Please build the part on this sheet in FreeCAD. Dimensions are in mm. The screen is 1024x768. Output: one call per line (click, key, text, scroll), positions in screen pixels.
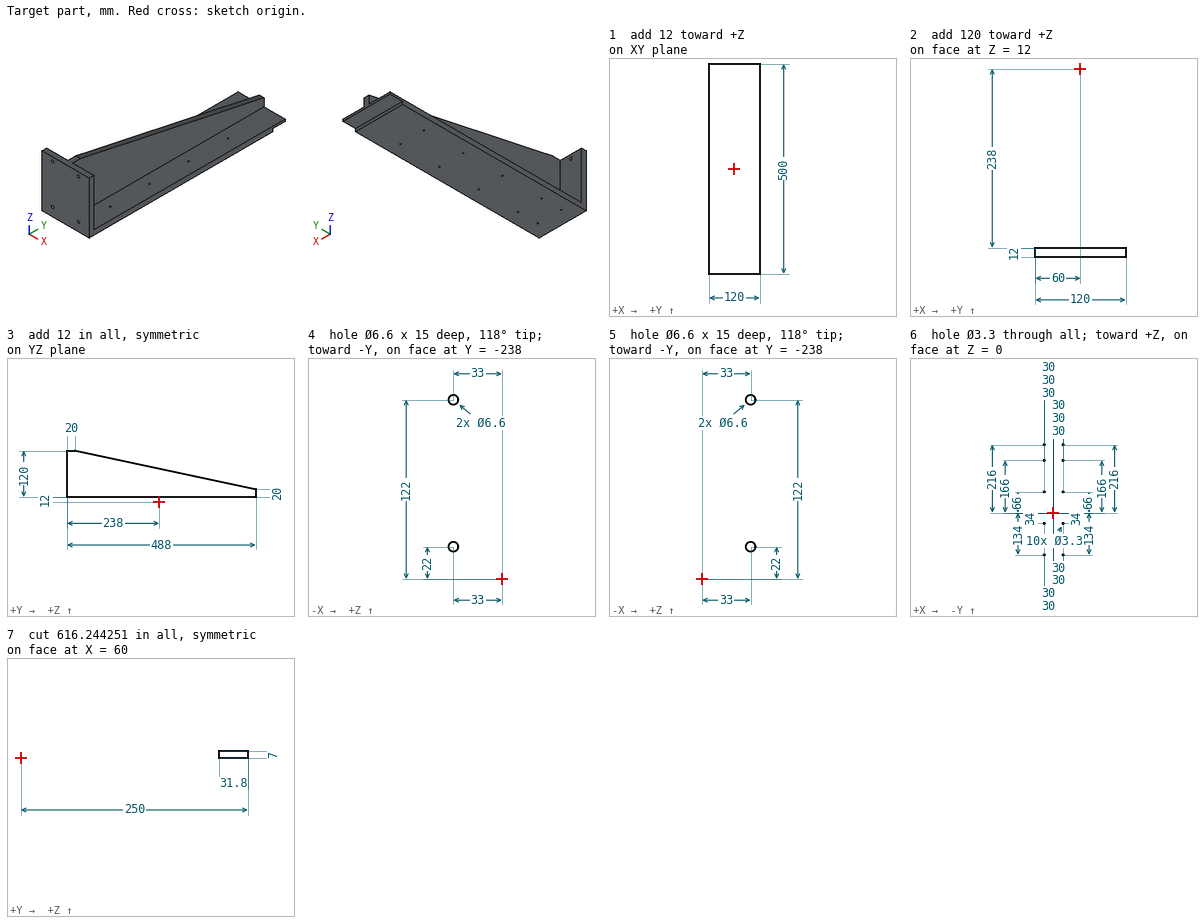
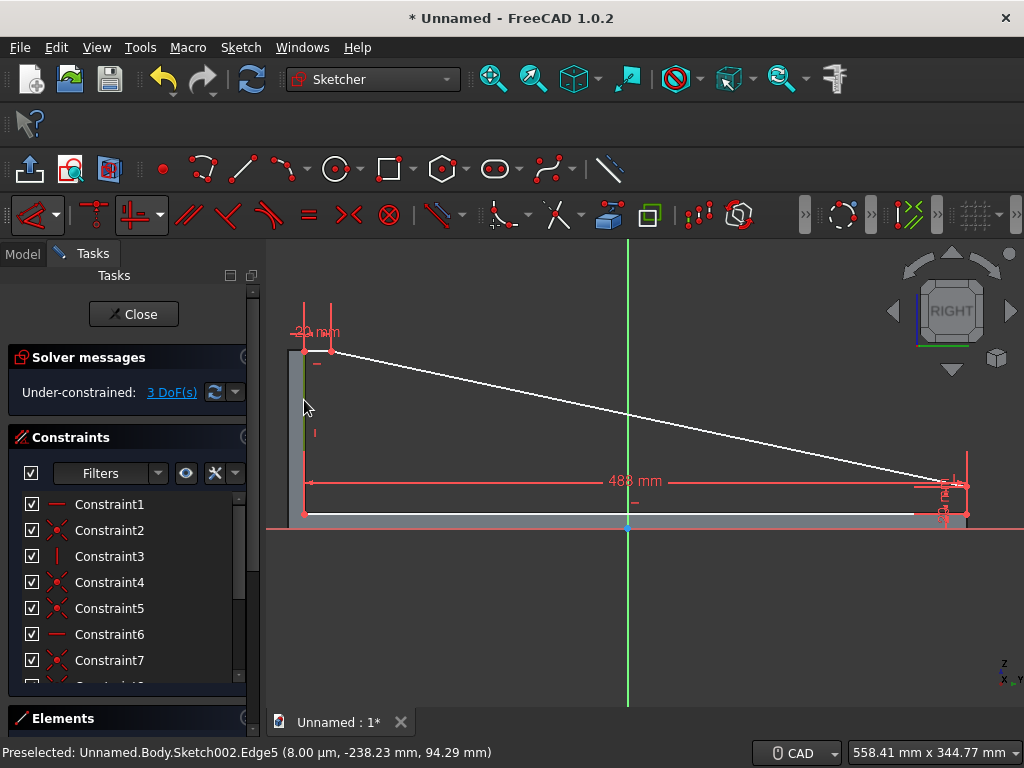
click(58, 216)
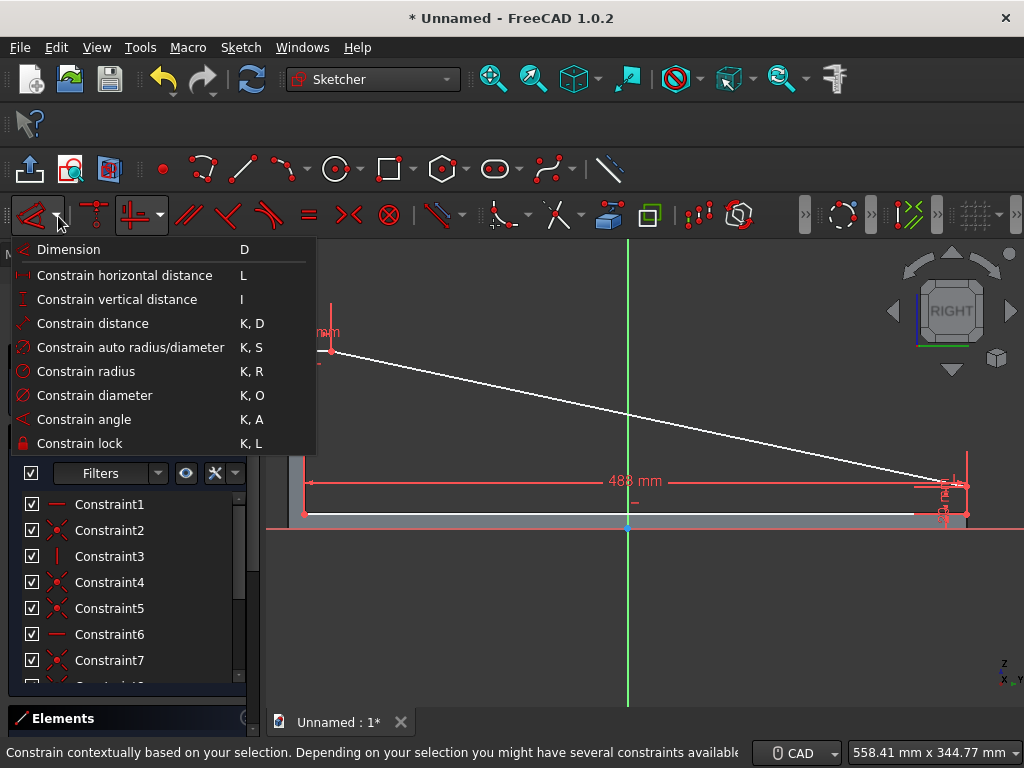
click(164, 299)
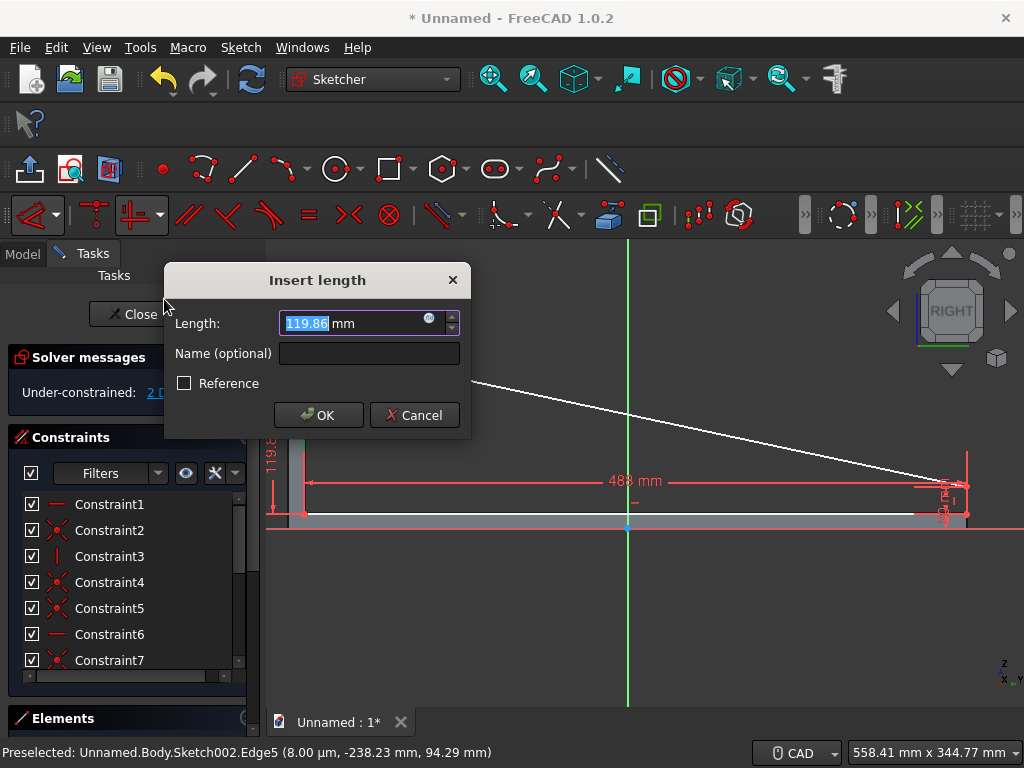
text(120)
key(Return)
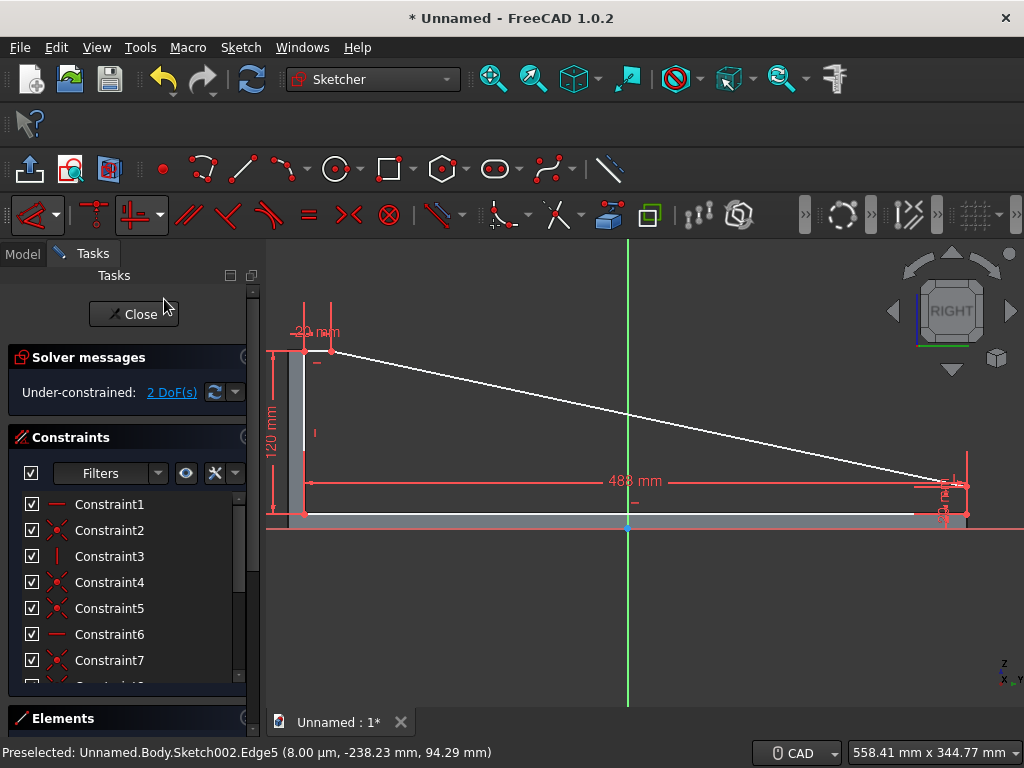
scroll(304, 514, up, 5)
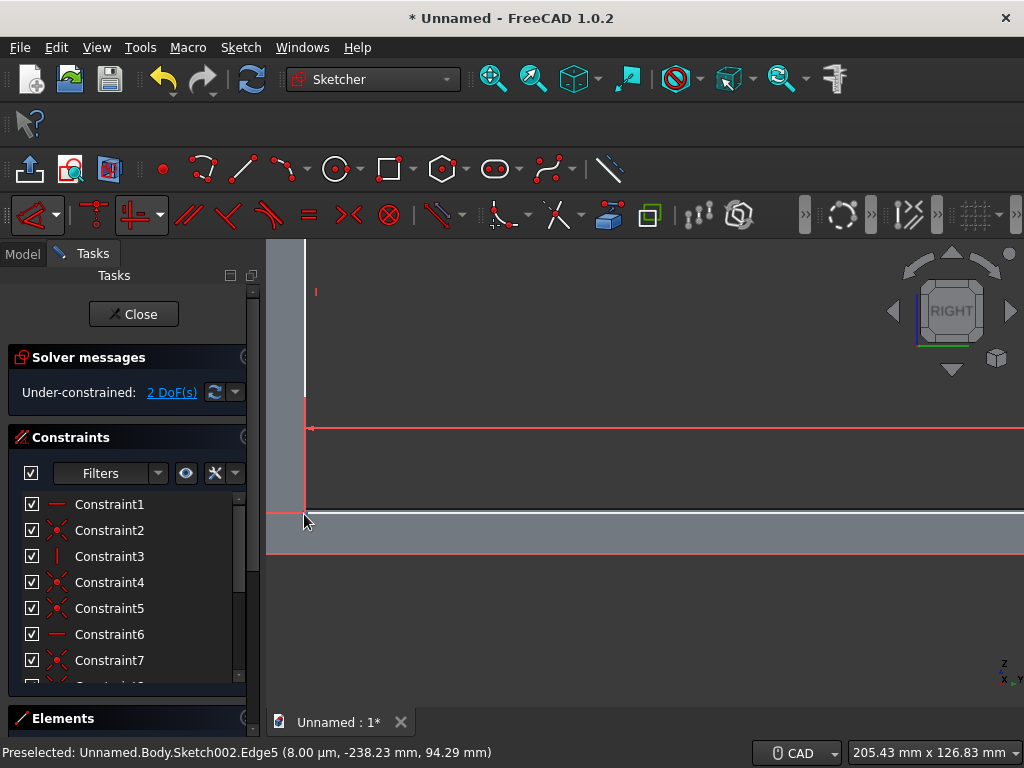
click(305, 513)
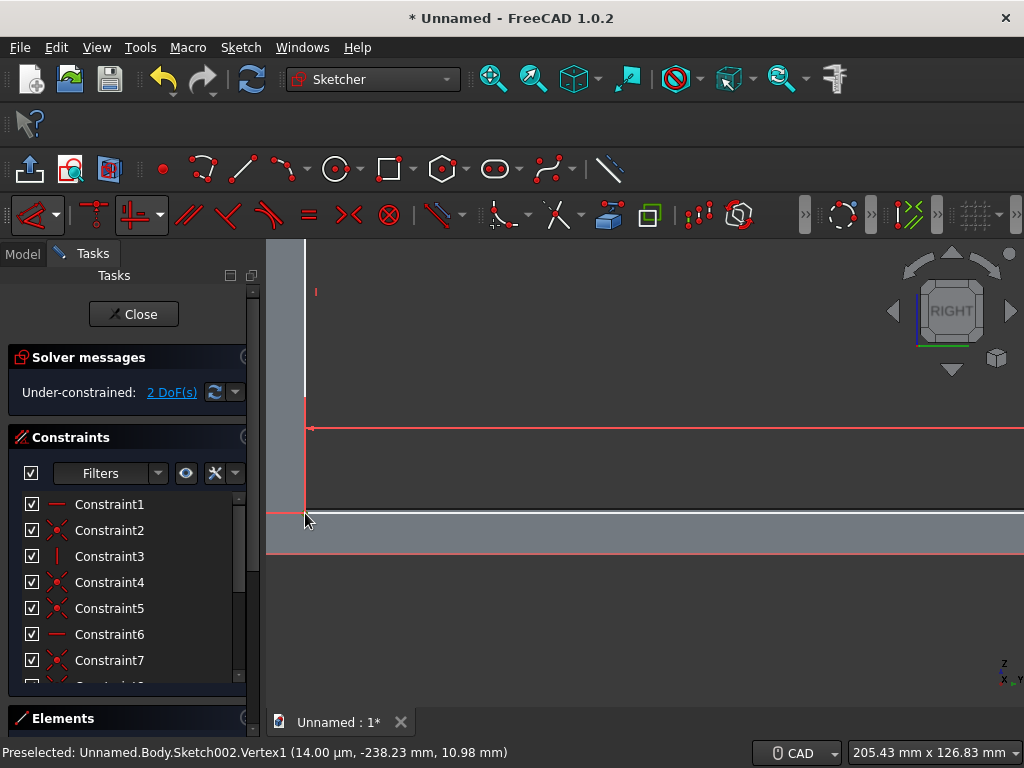
click(58, 216)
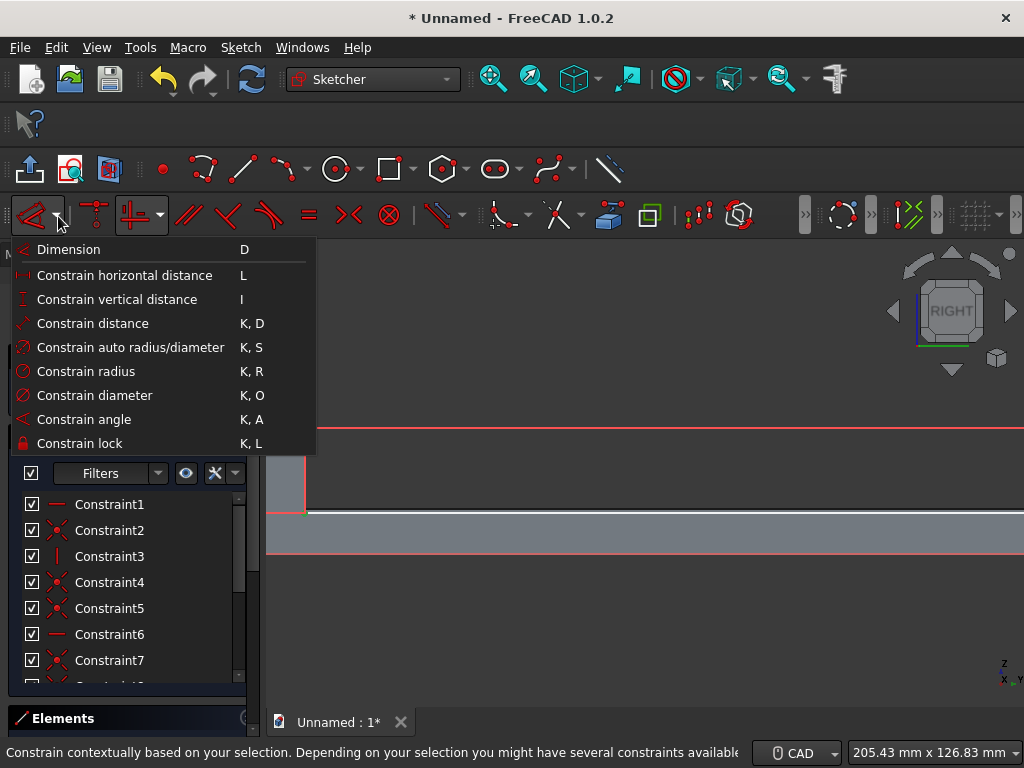
click(164, 299)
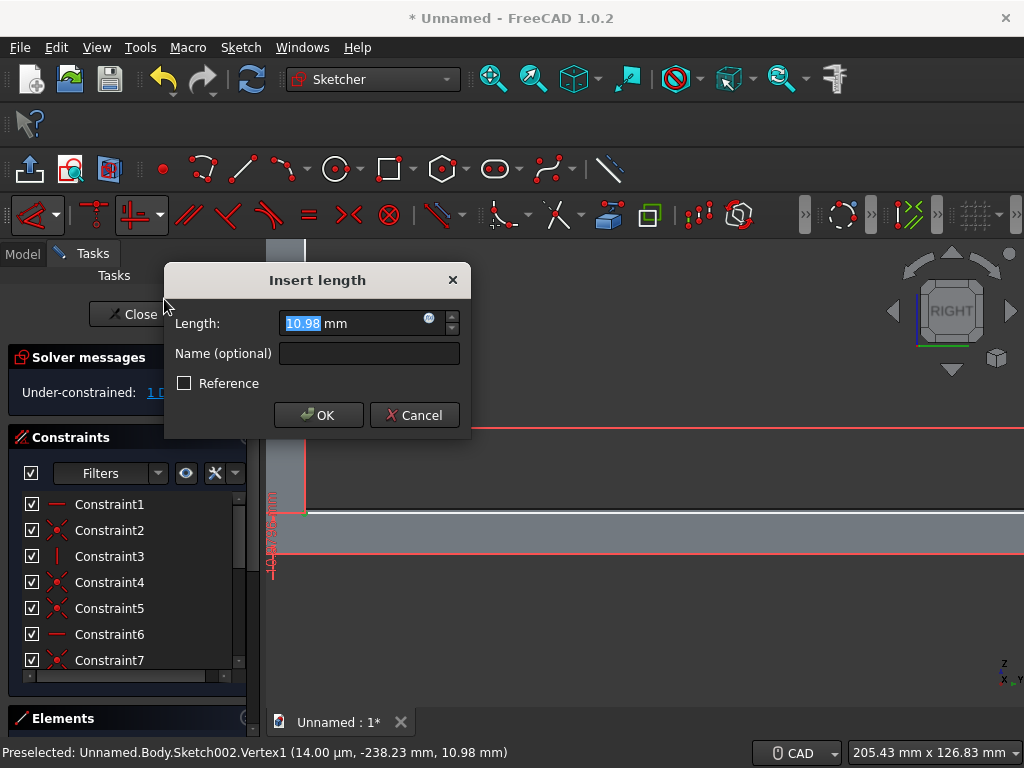
text(12)
key(Return)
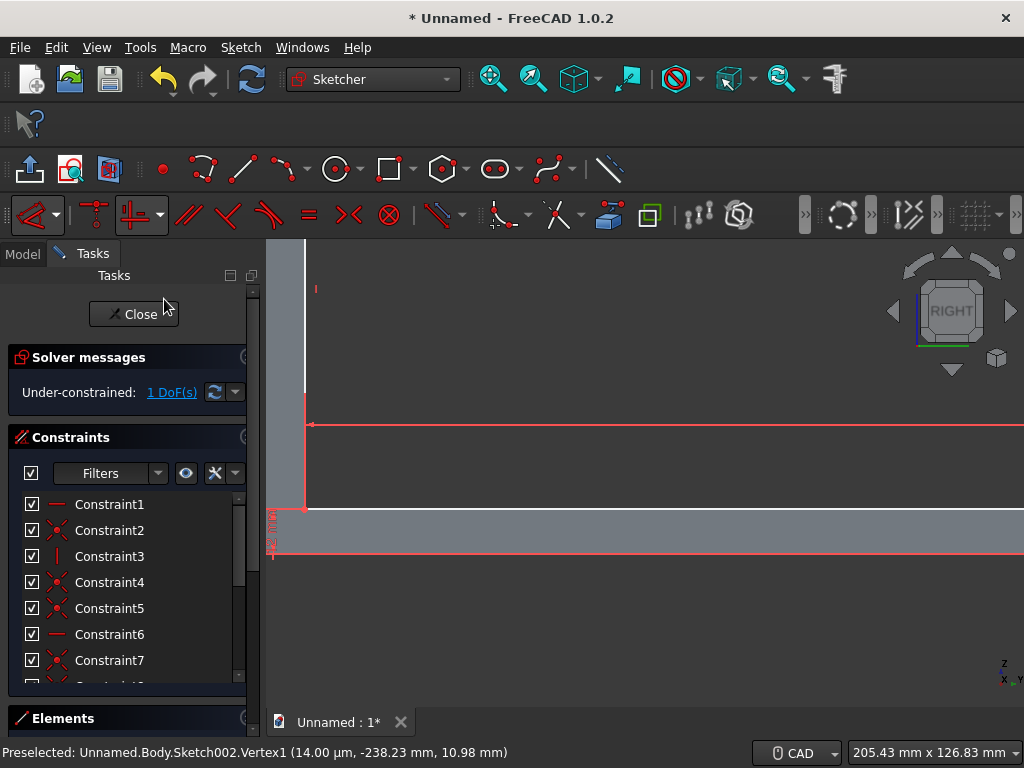
scroll(417, 514, down, 8)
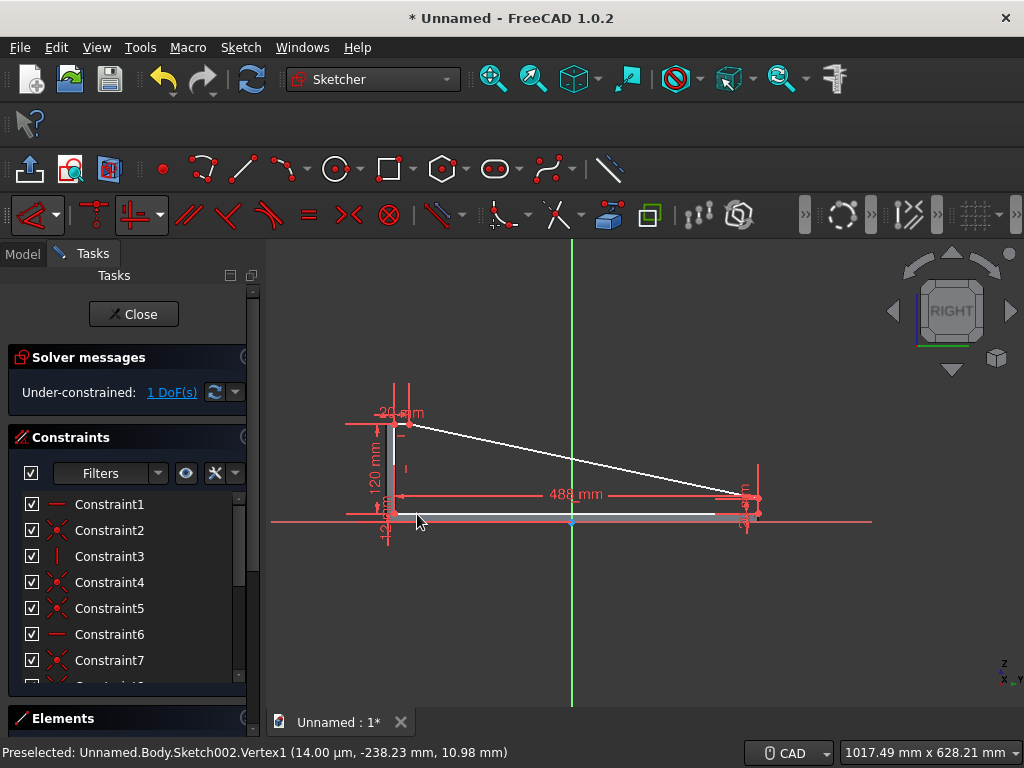
click(394, 514)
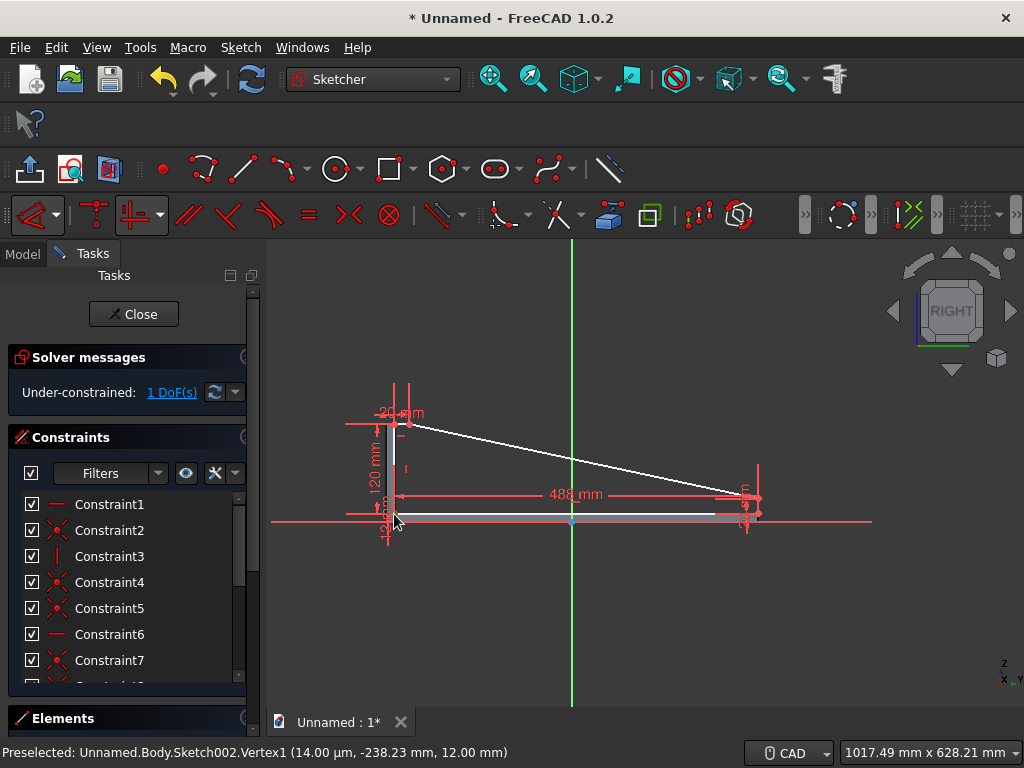
click(58, 216)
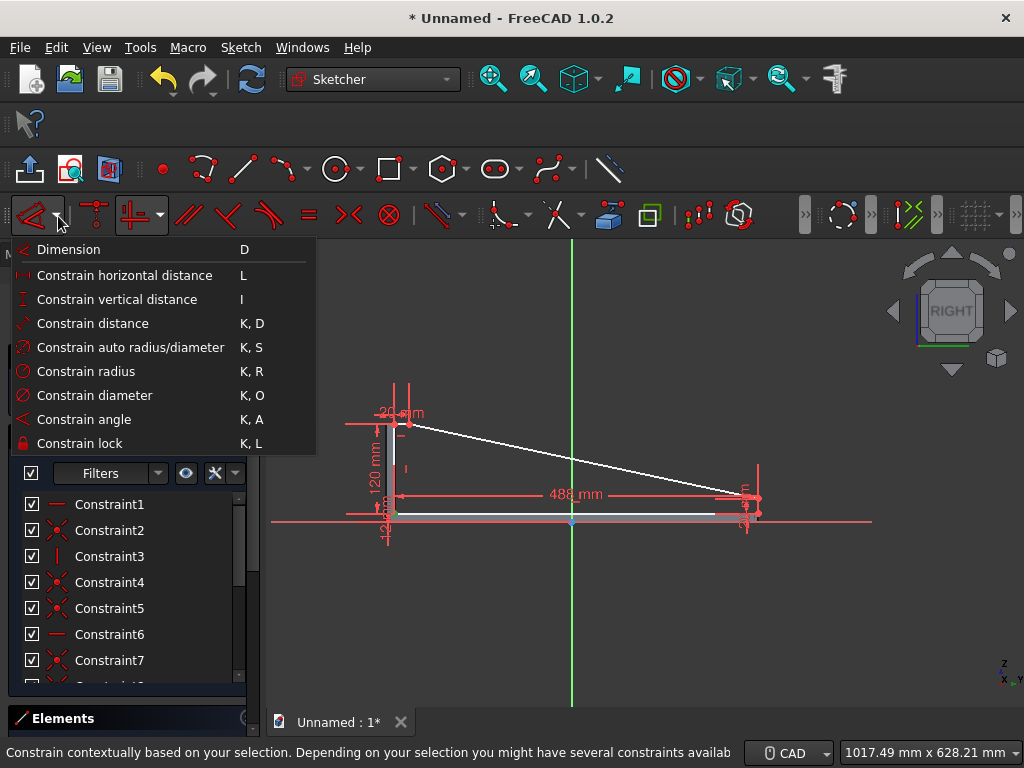
click(164, 275)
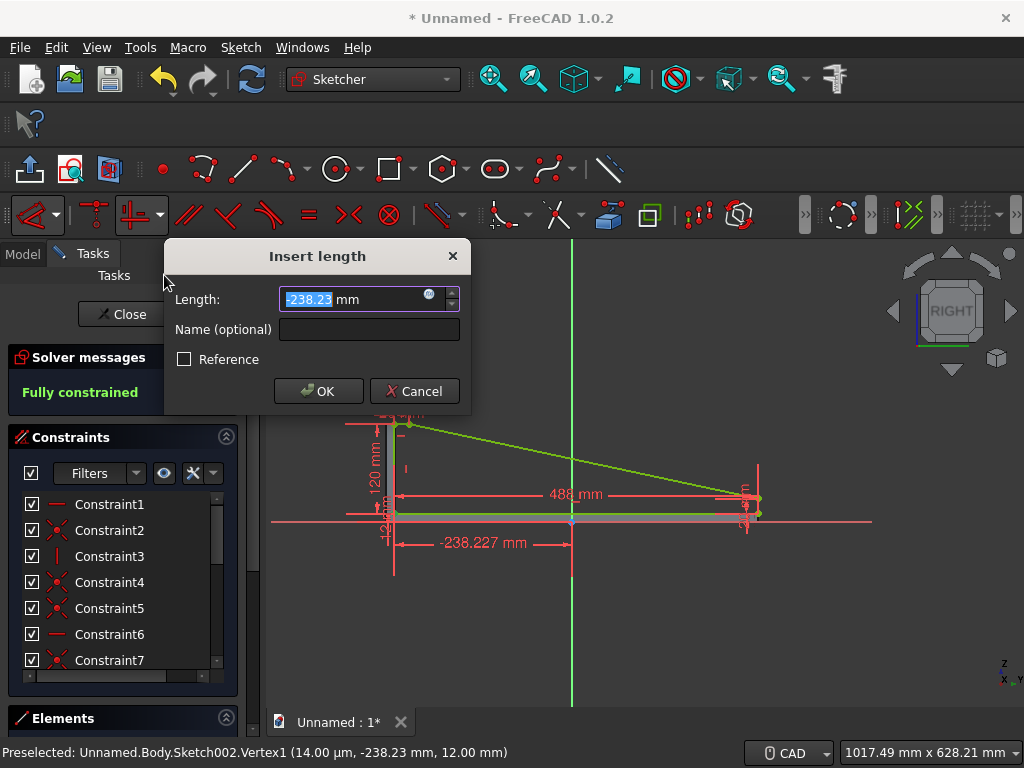
text(-238)
key(Return)